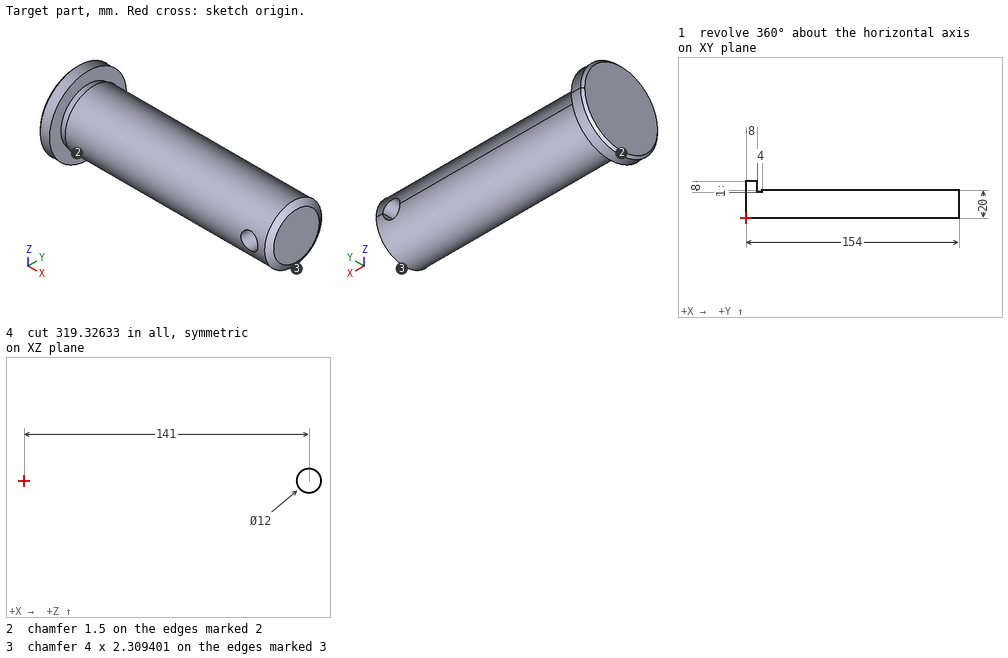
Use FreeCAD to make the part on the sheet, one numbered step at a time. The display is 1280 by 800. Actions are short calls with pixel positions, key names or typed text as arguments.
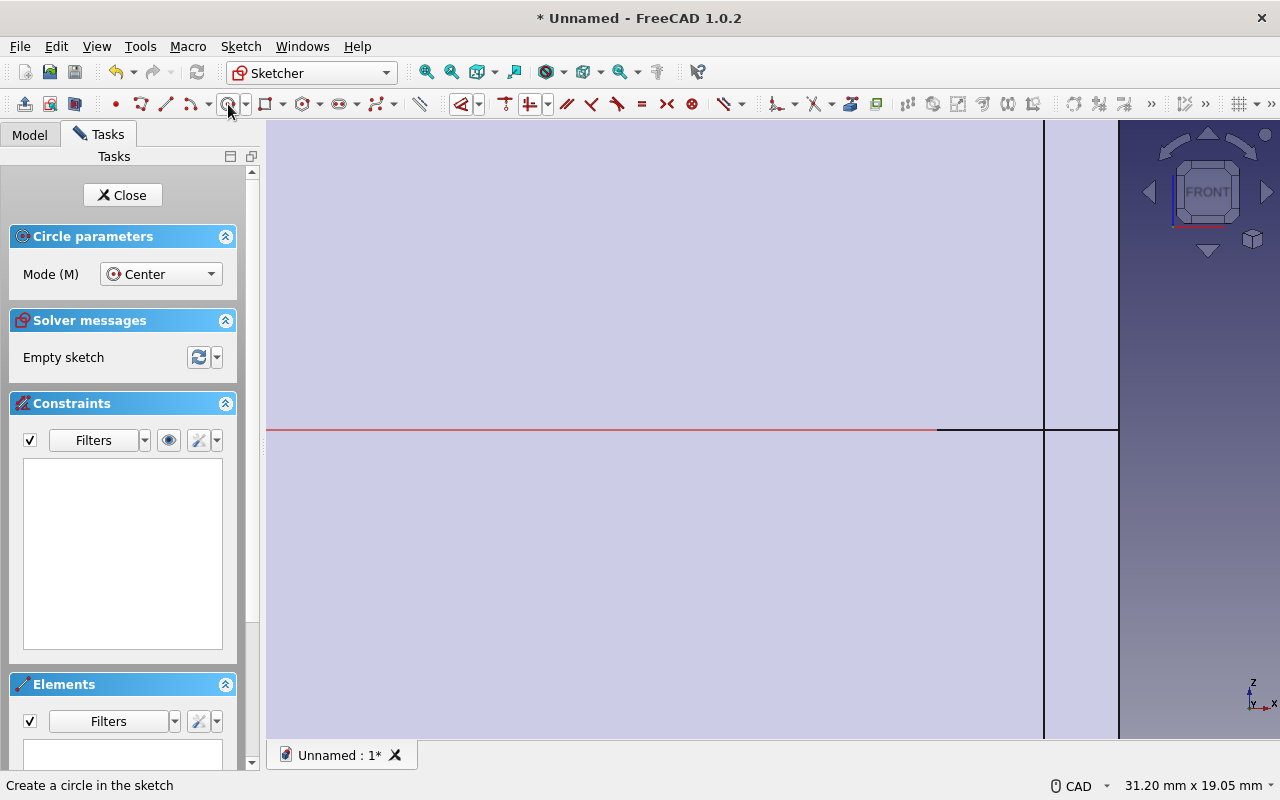
click(696, 429)
move(834, 292)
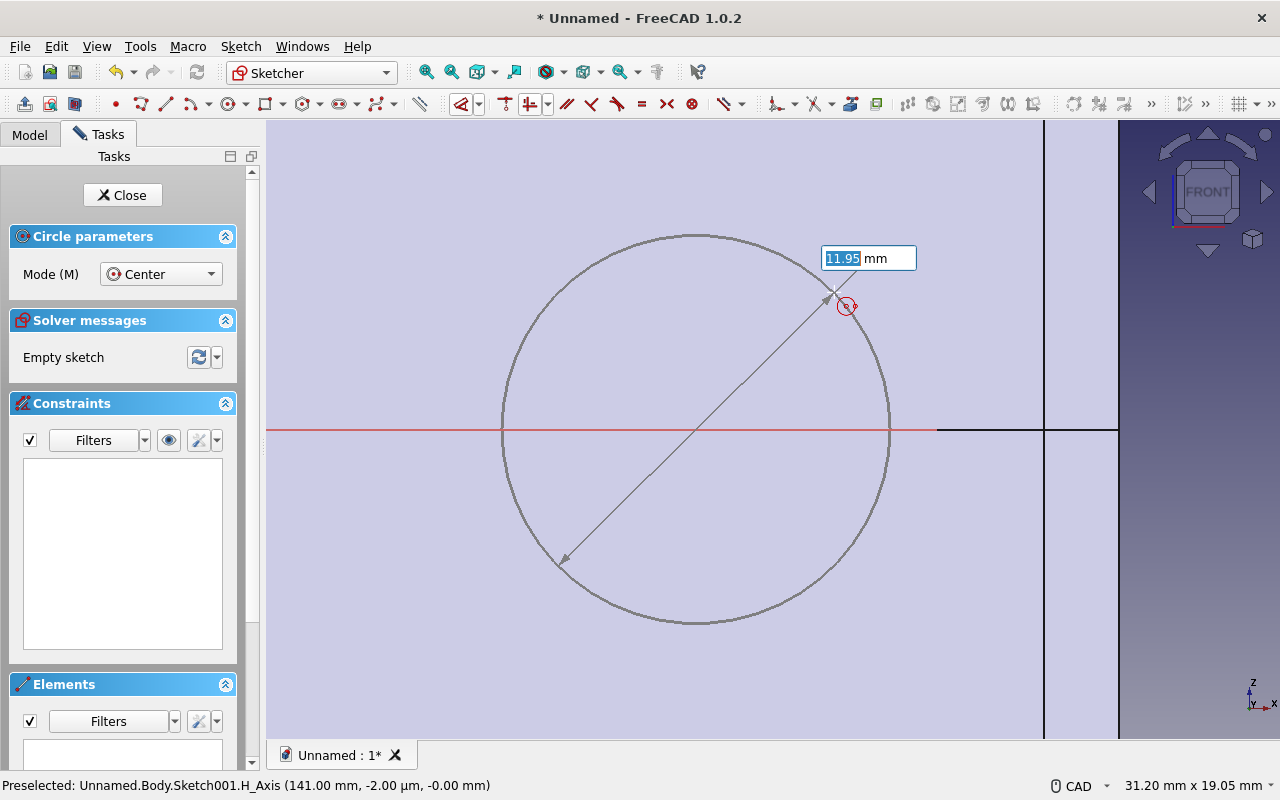
text(12)
key(Return)
key(Escape)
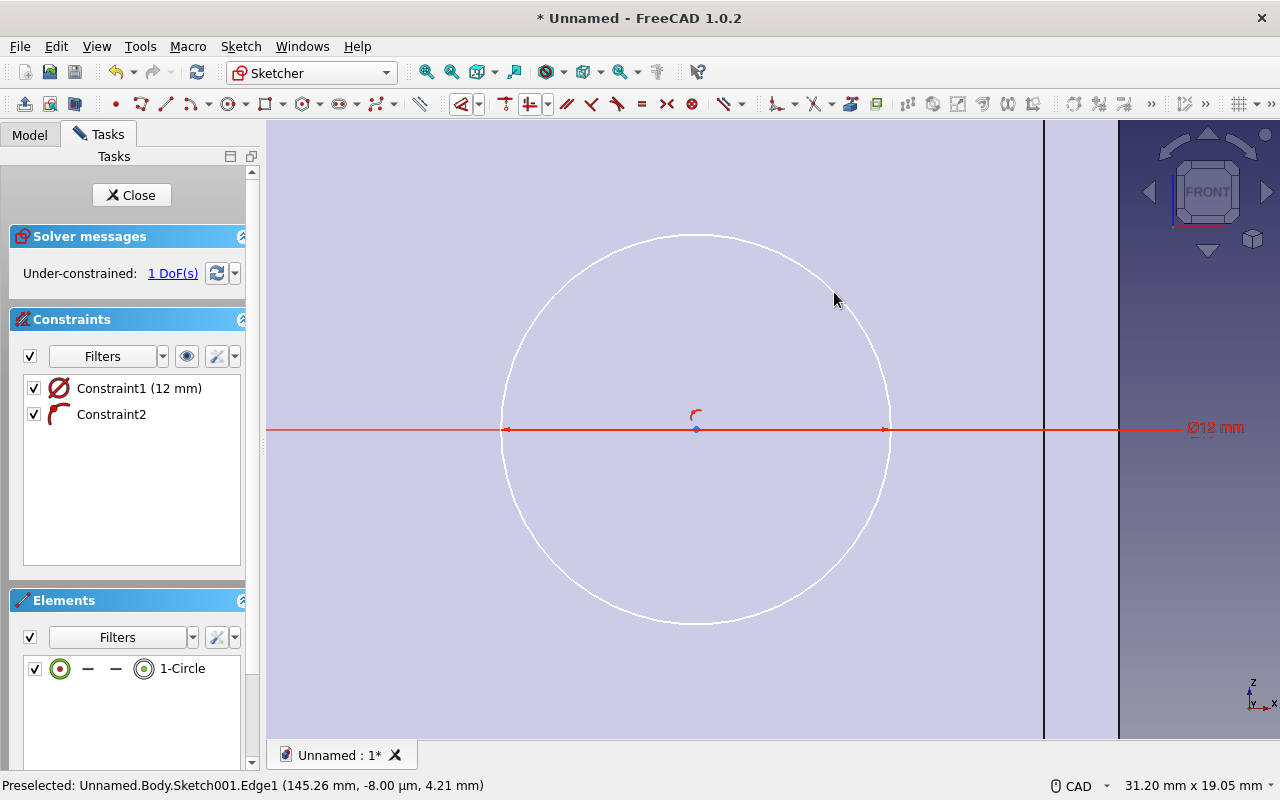
click(696, 429)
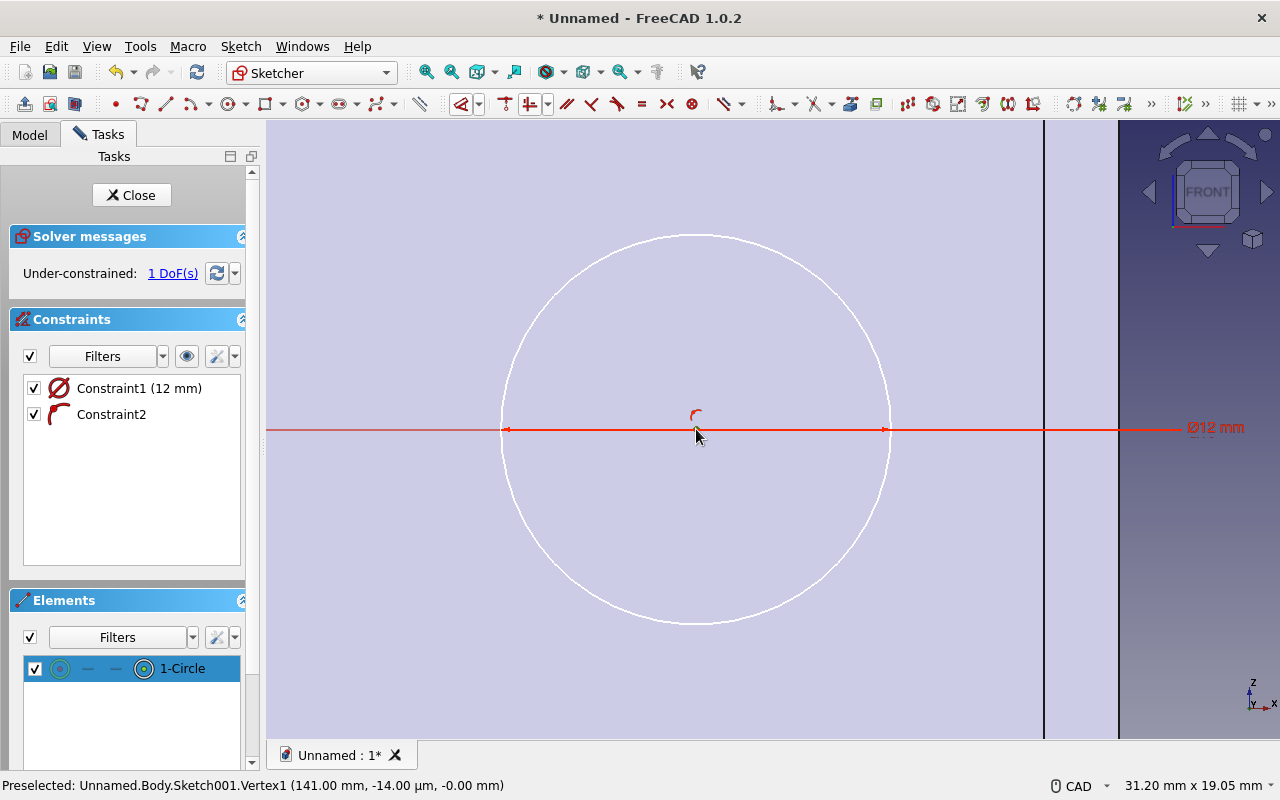
key(l)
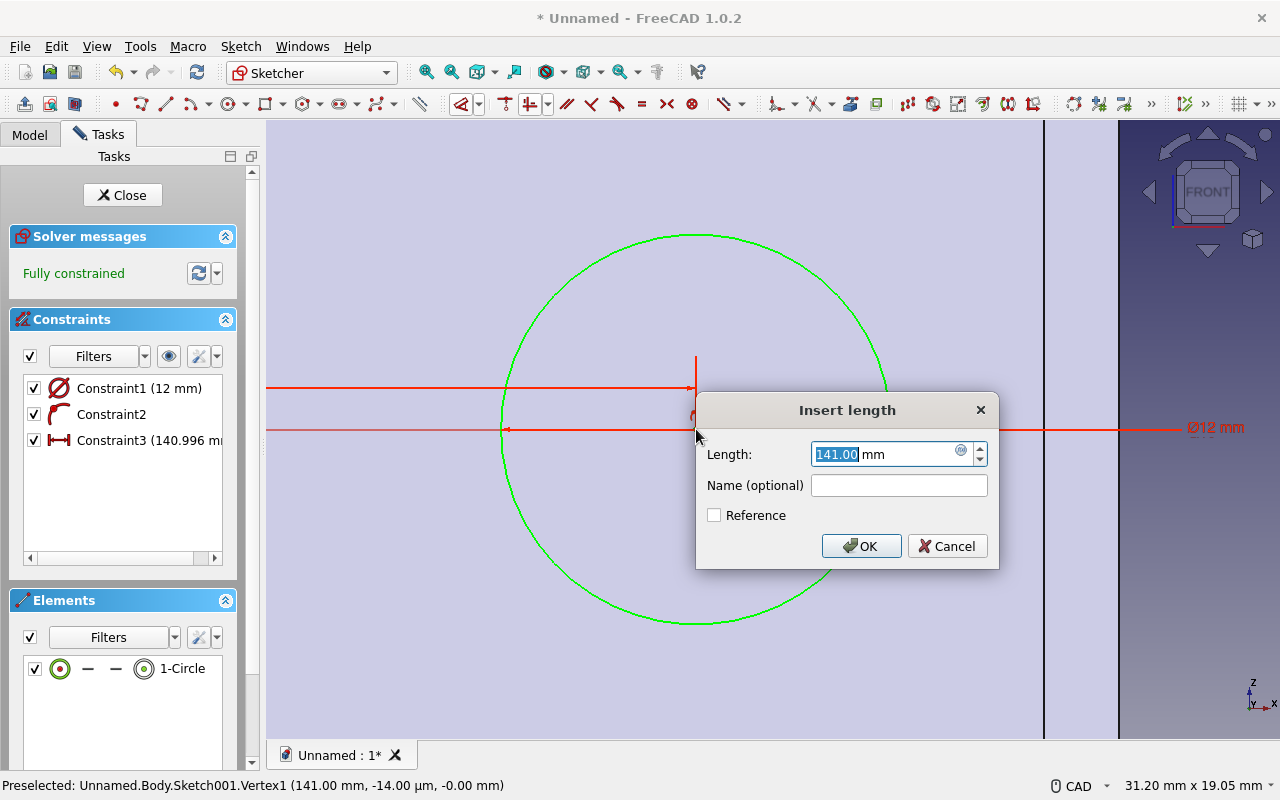
text(141)
key(Return)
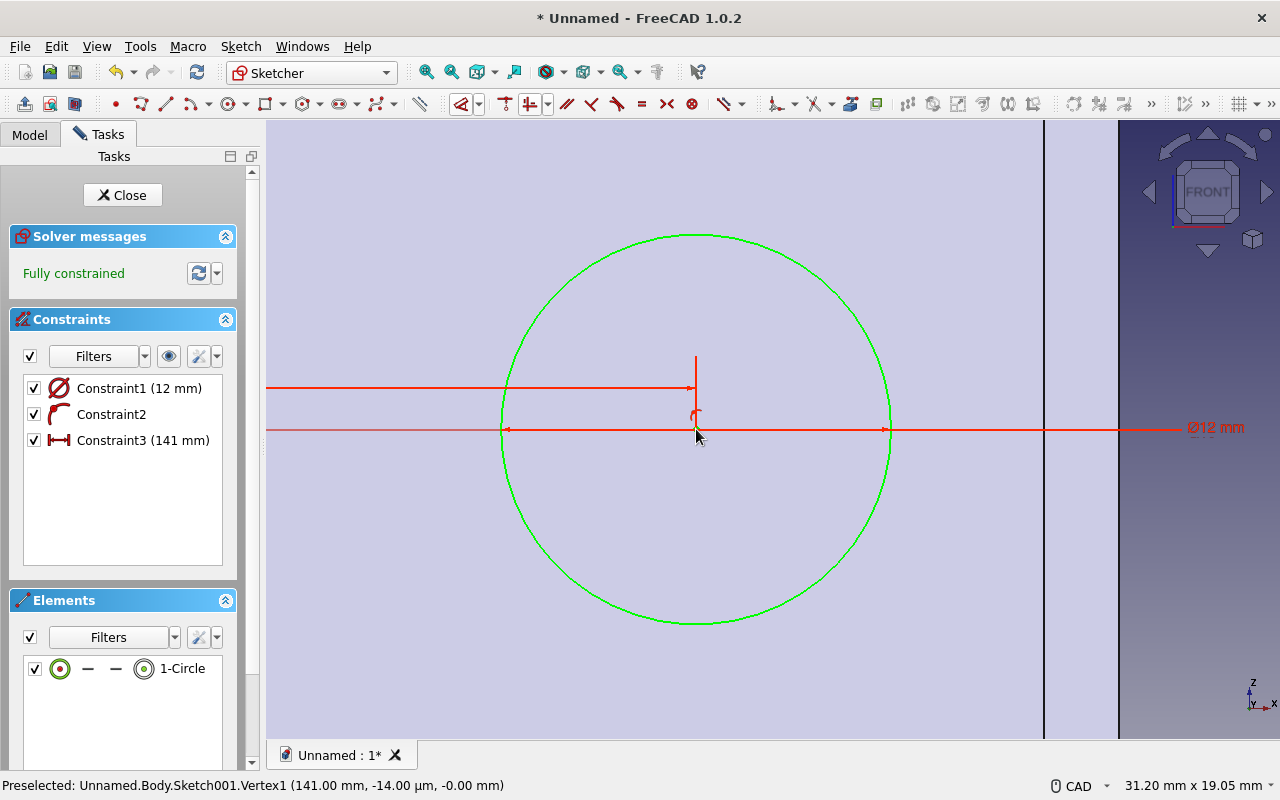
click(123, 195)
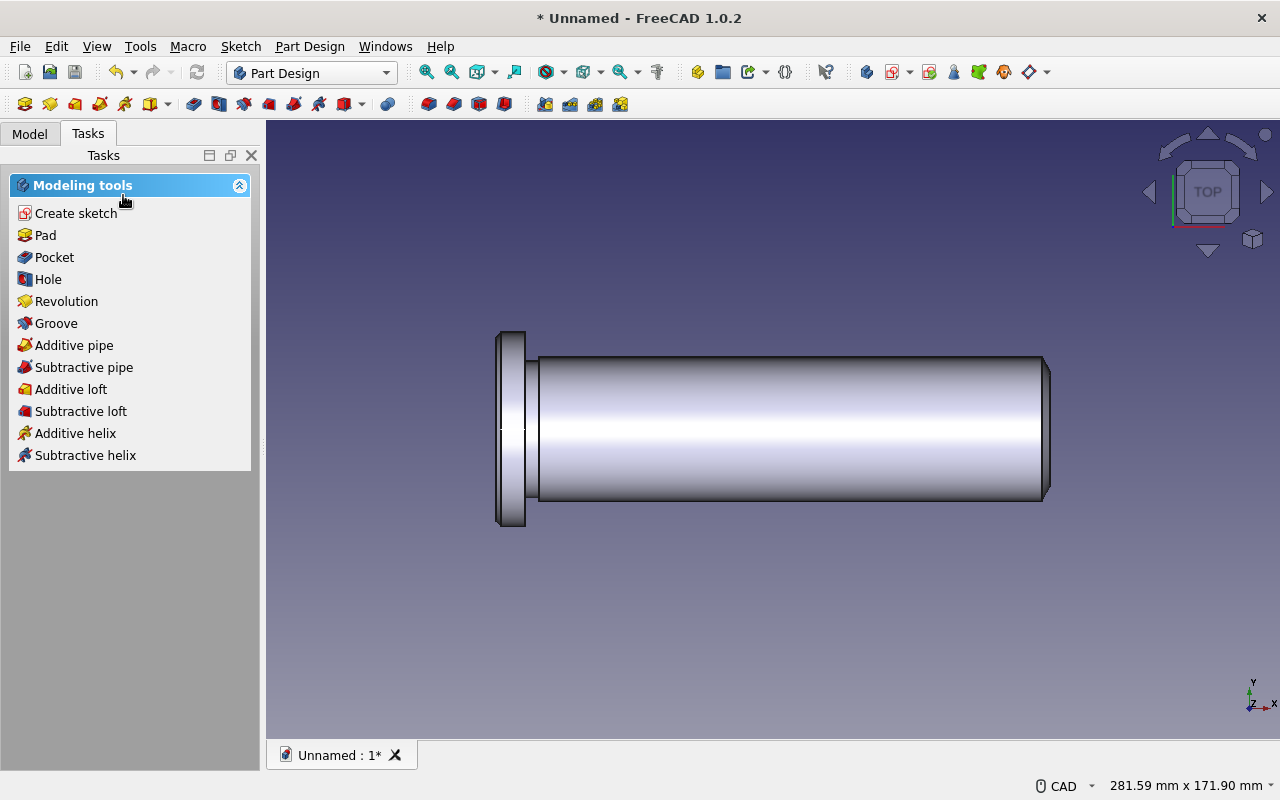
click(194, 104)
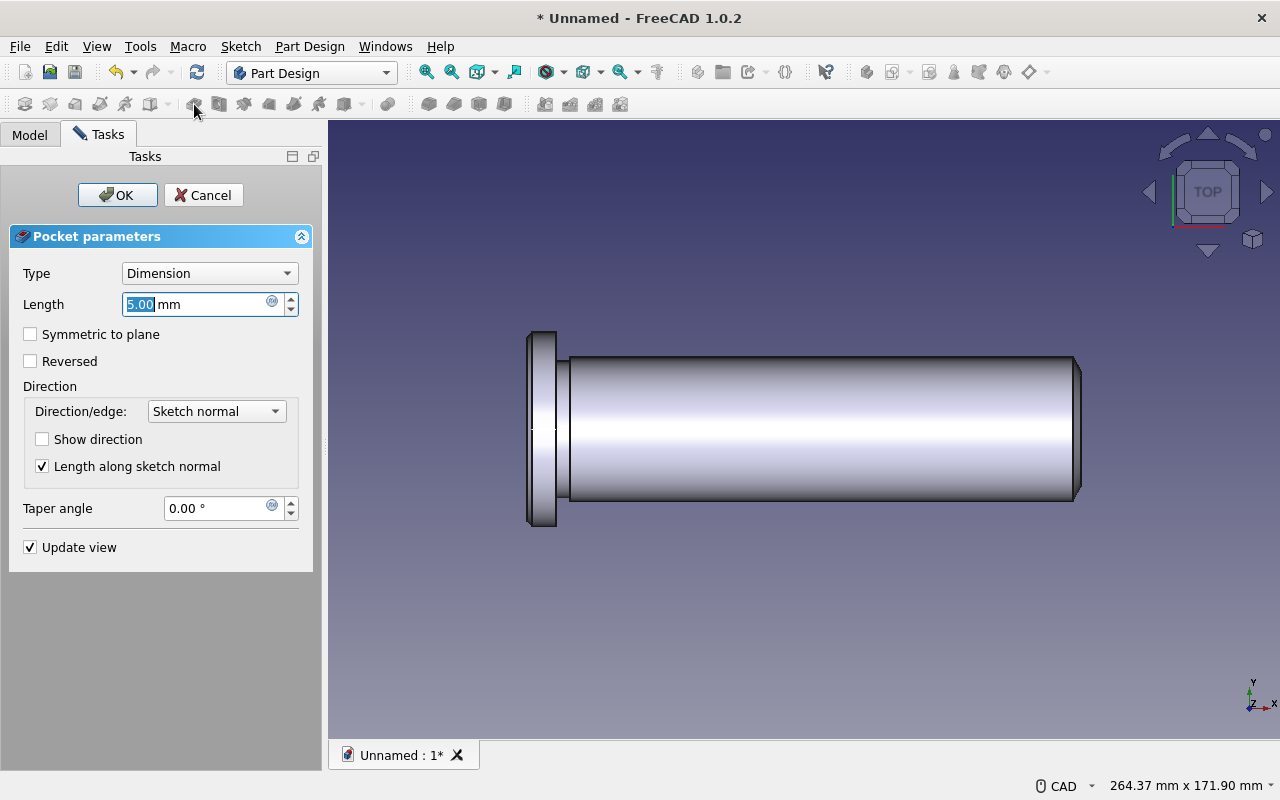
text(319.32633)
key(Tab)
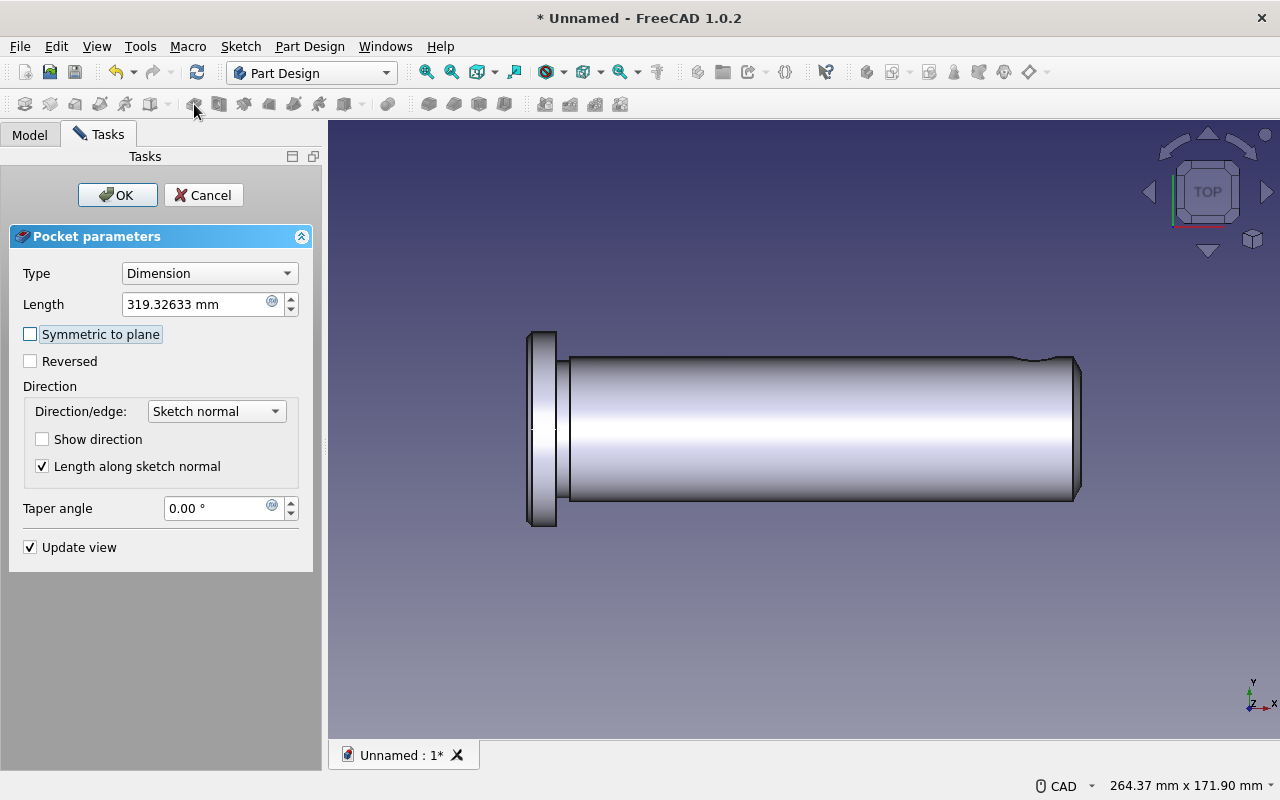
click(31, 334)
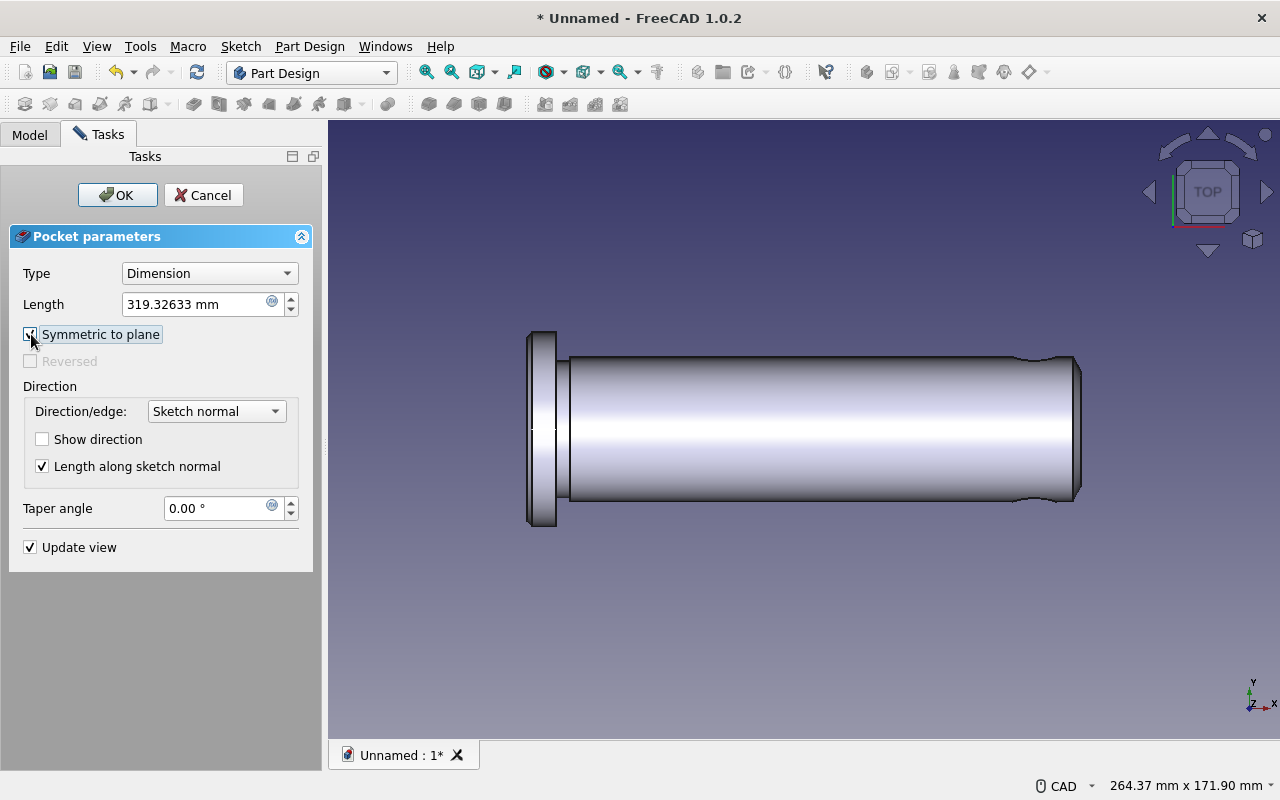
click(118, 195)